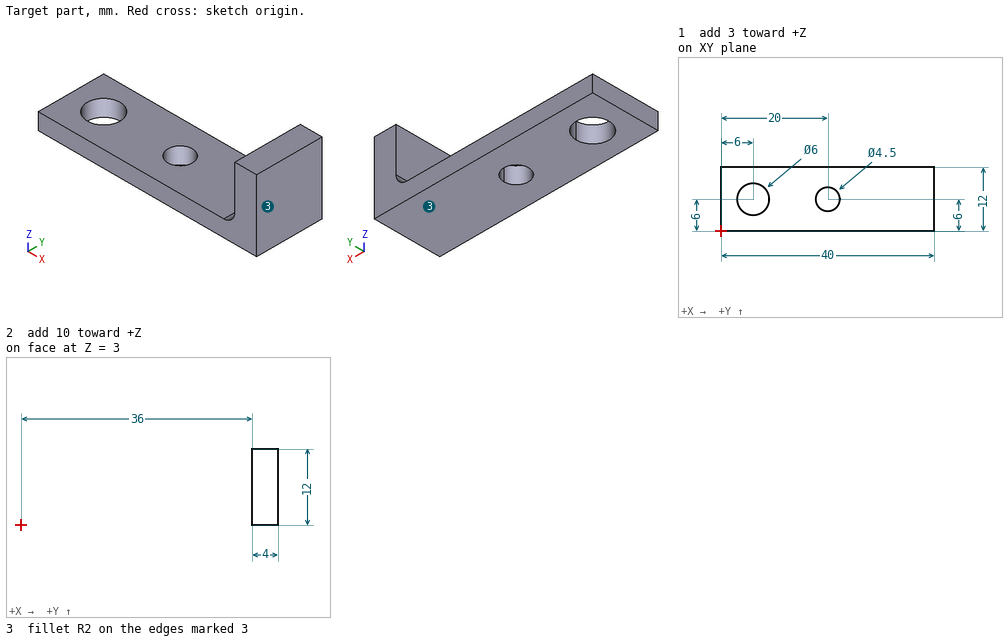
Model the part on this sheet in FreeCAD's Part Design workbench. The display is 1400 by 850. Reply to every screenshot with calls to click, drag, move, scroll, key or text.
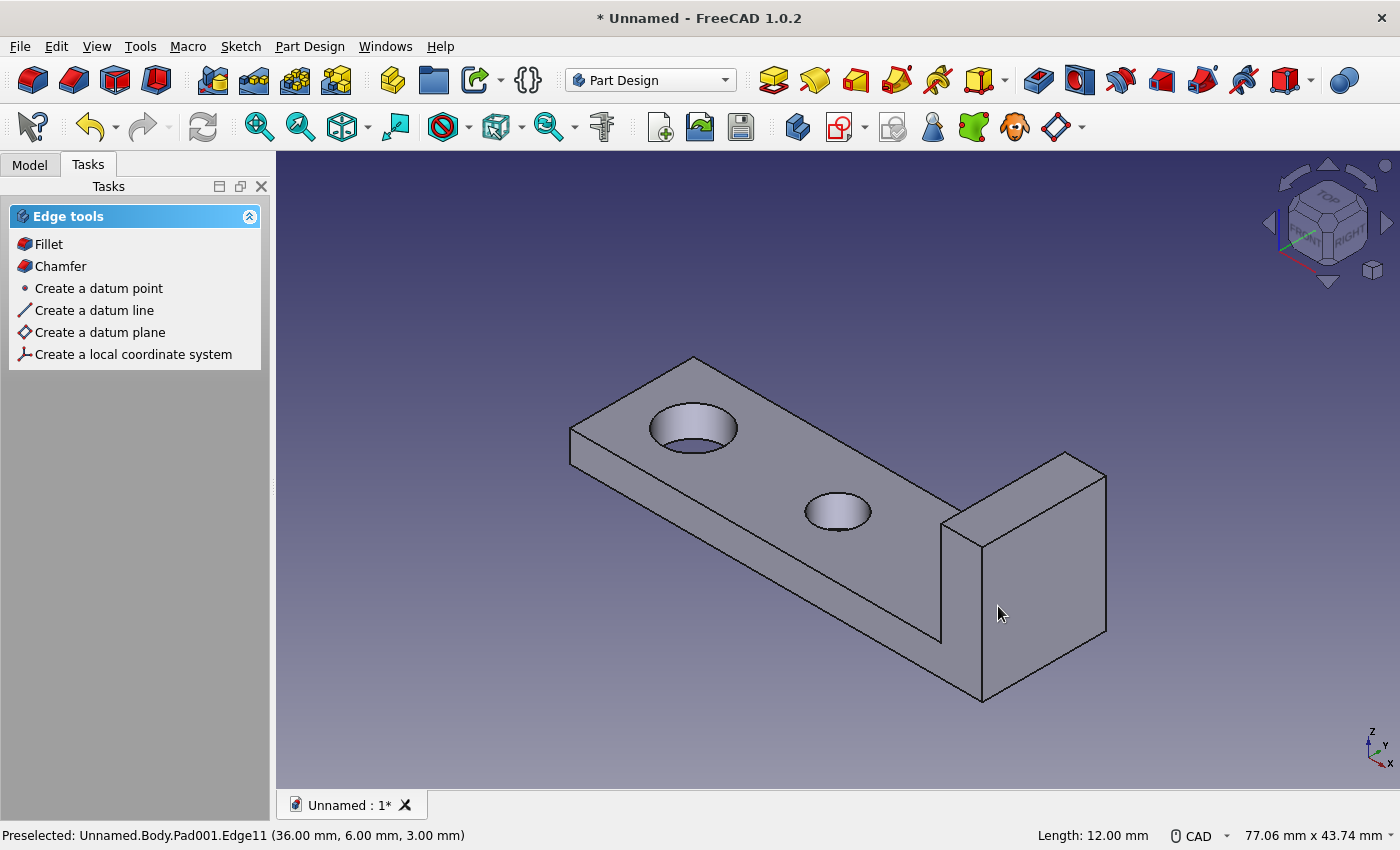
click(33, 80)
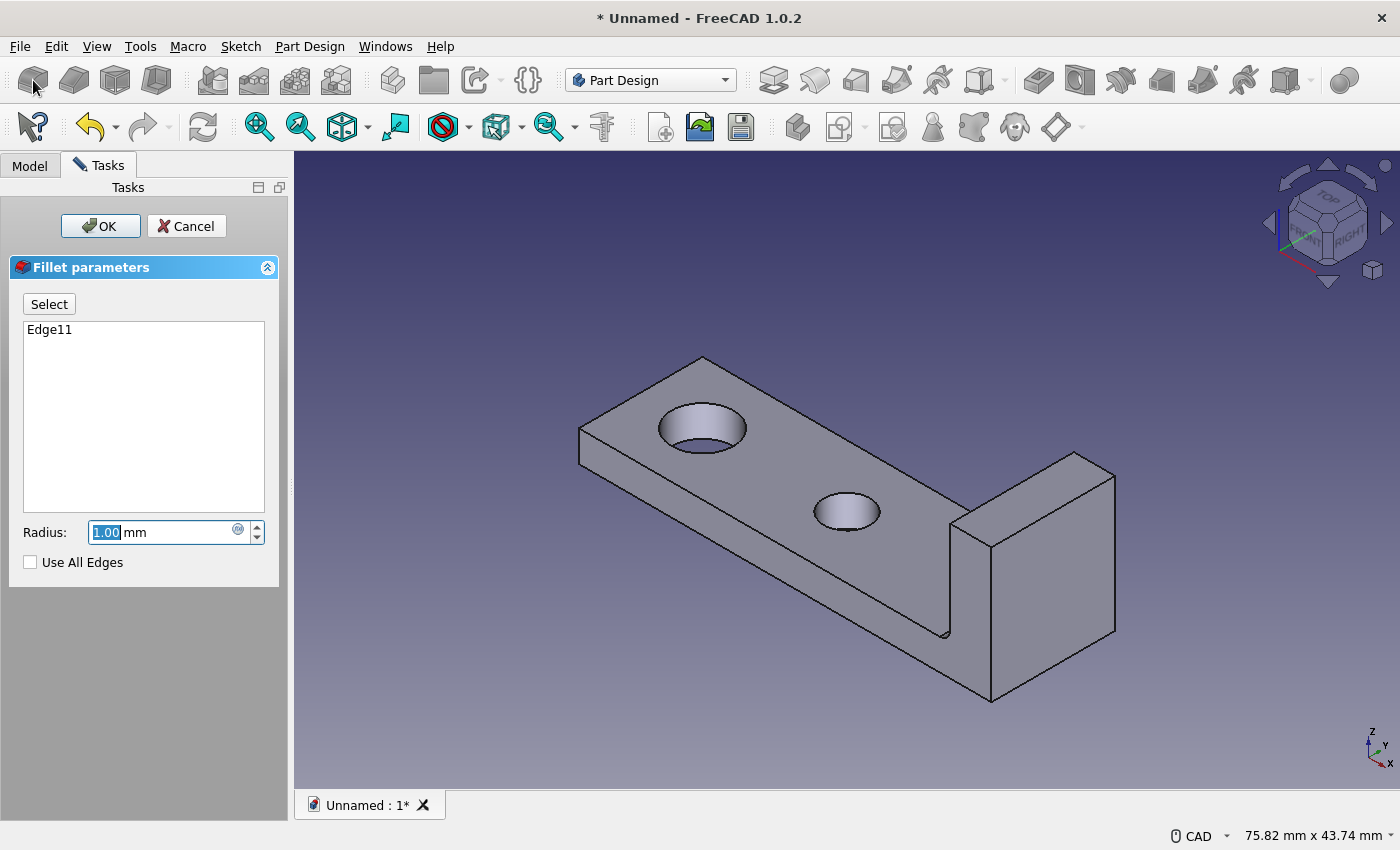
text(2)
key(Tab)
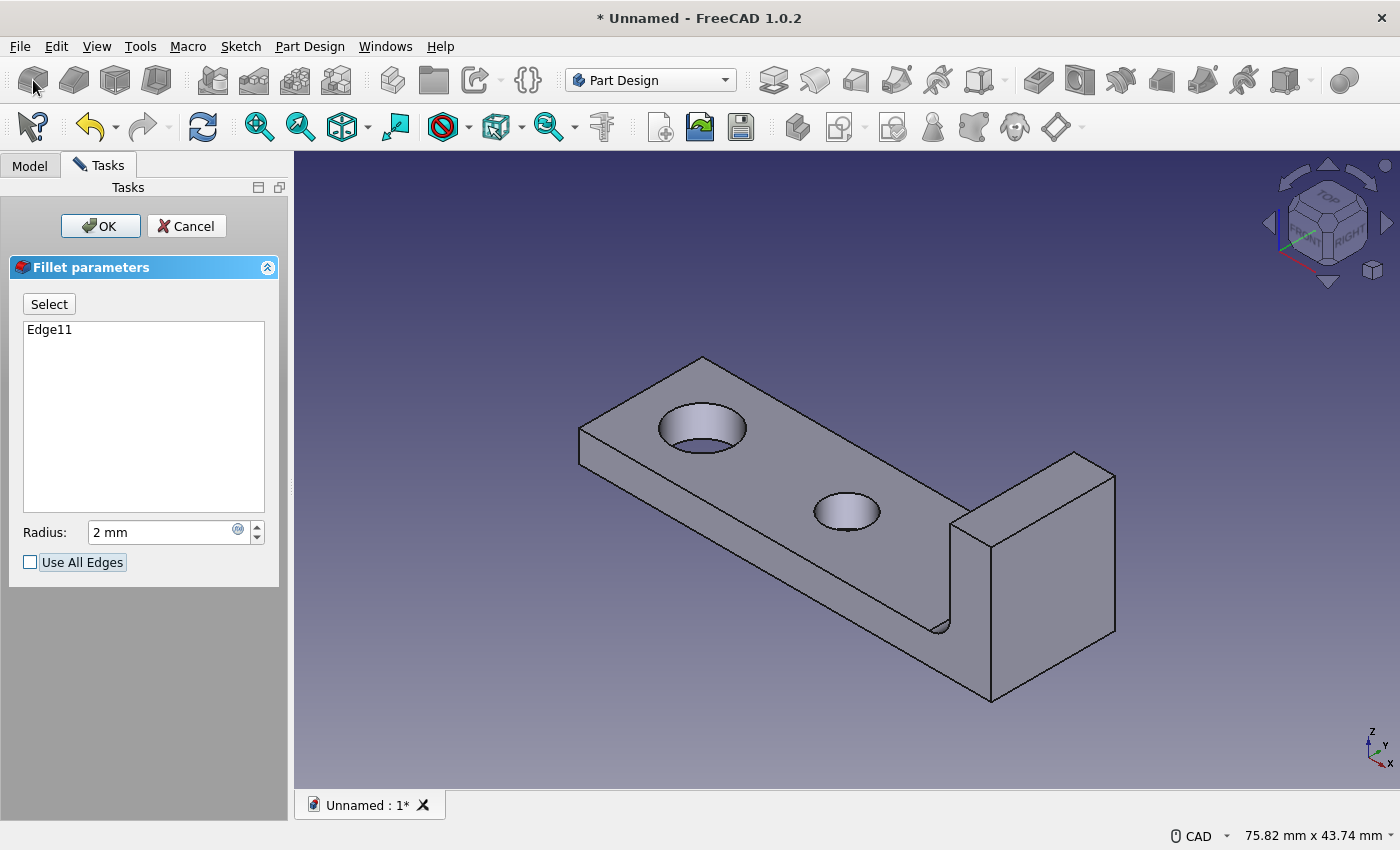
click(101, 226)